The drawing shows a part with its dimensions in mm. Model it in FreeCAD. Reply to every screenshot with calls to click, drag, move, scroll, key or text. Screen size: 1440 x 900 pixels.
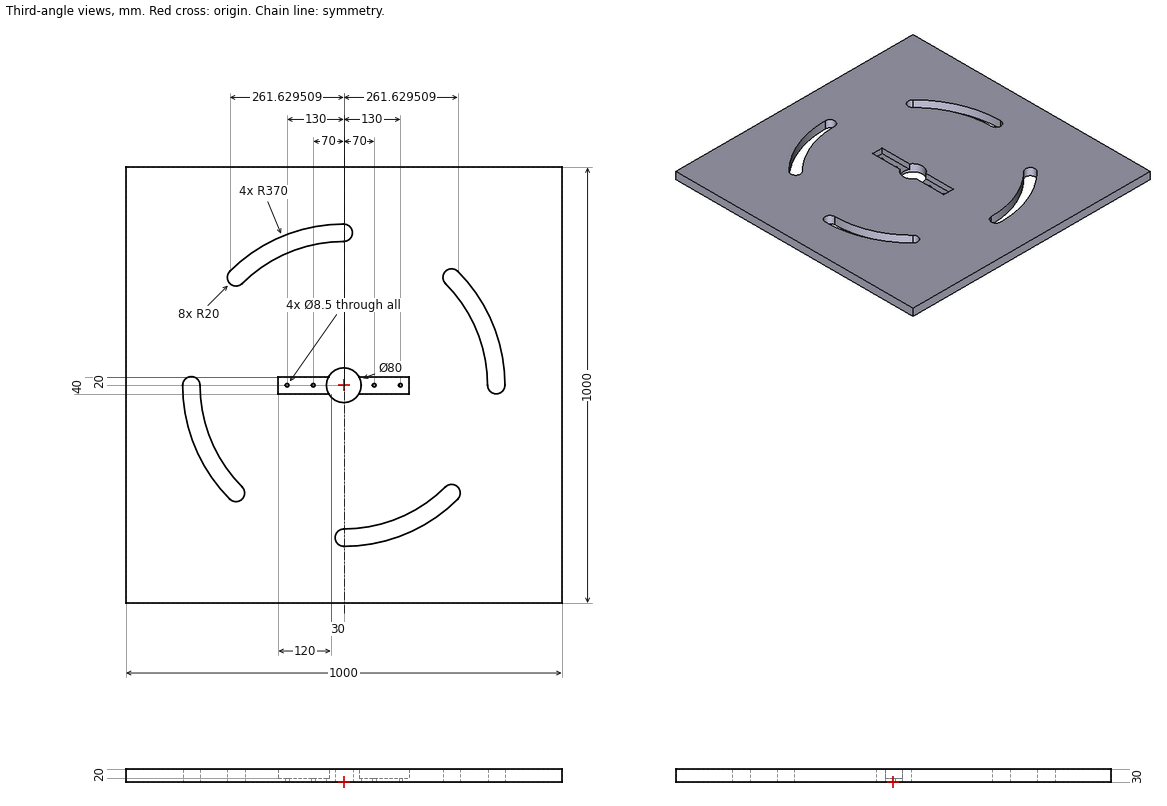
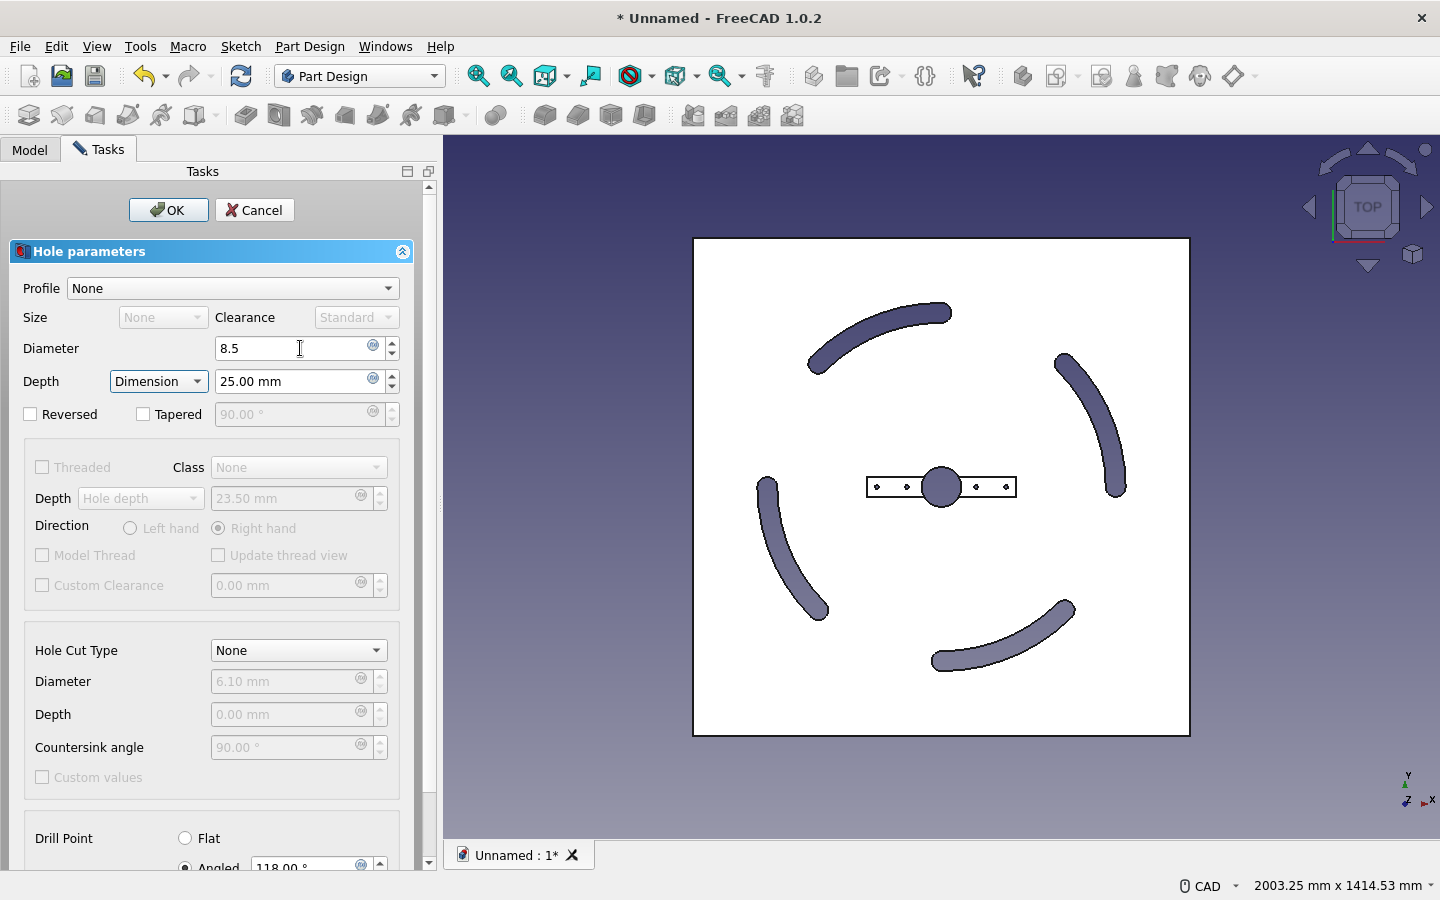
click(160, 382)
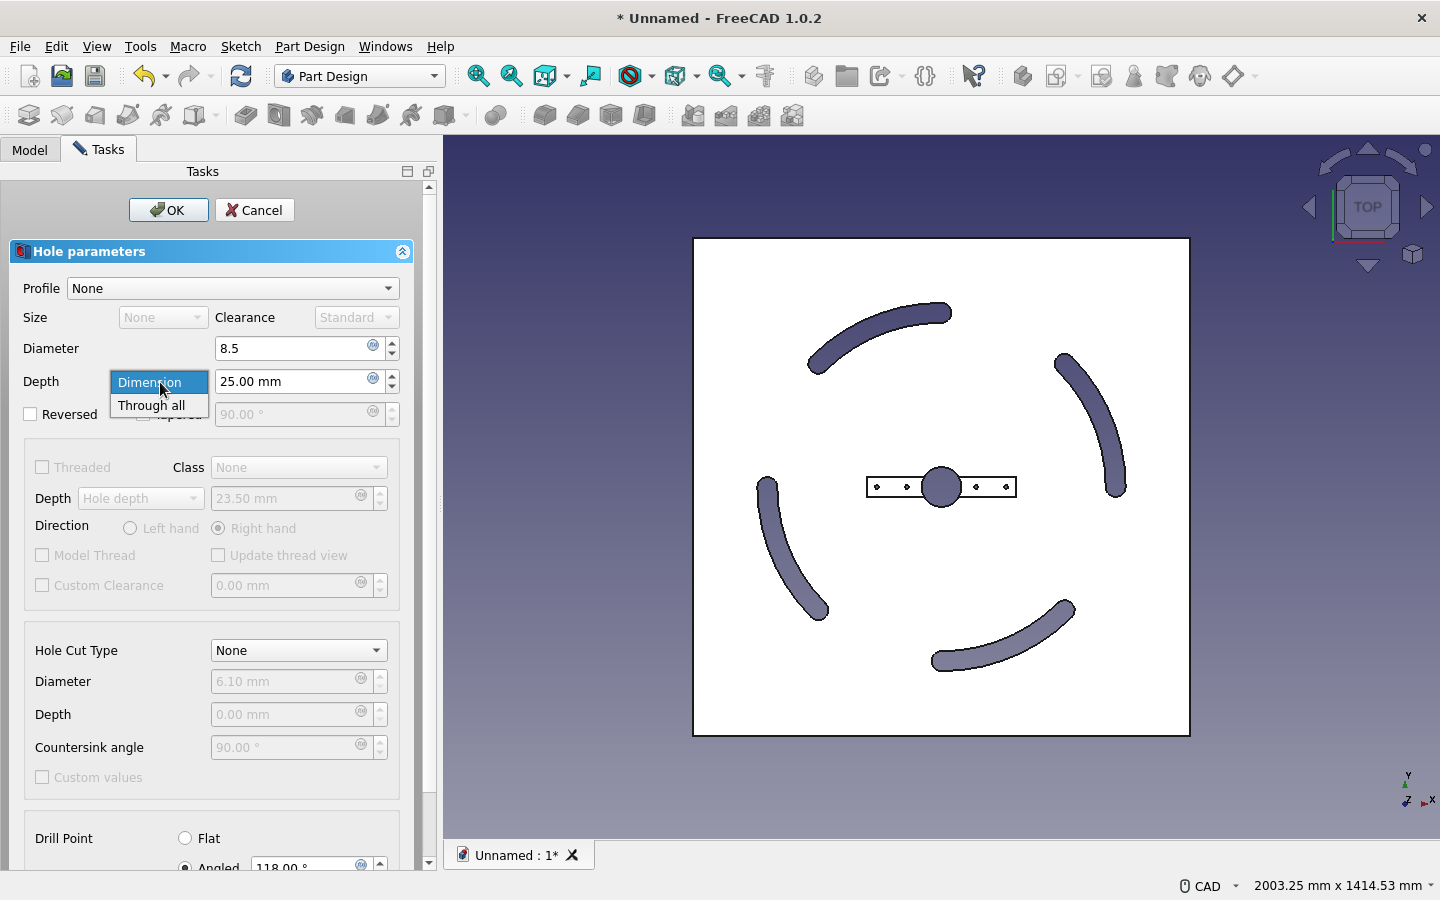
click(158, 406)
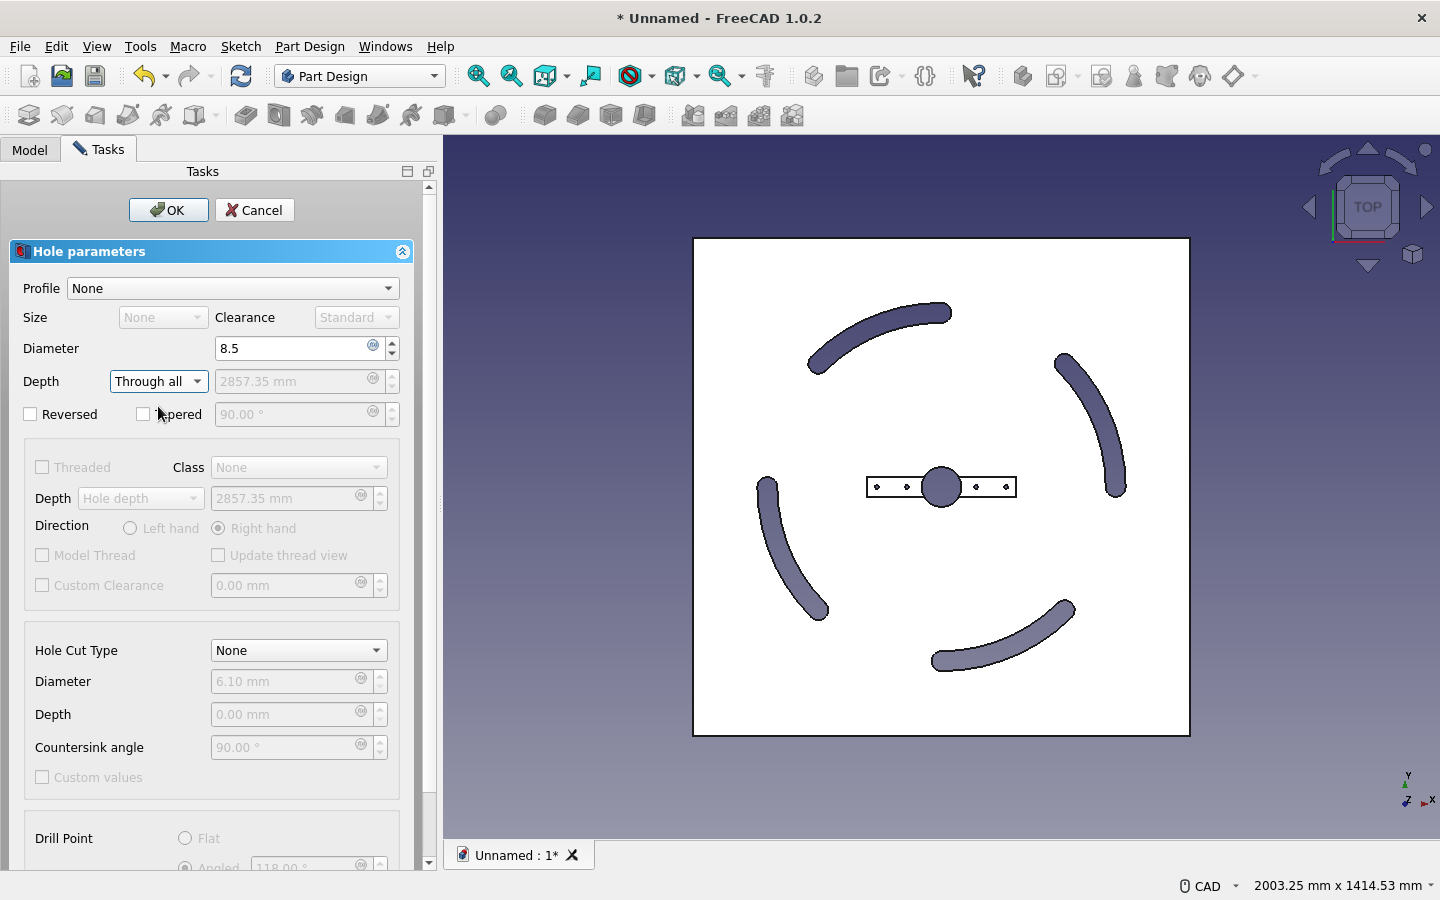
click(169, 210)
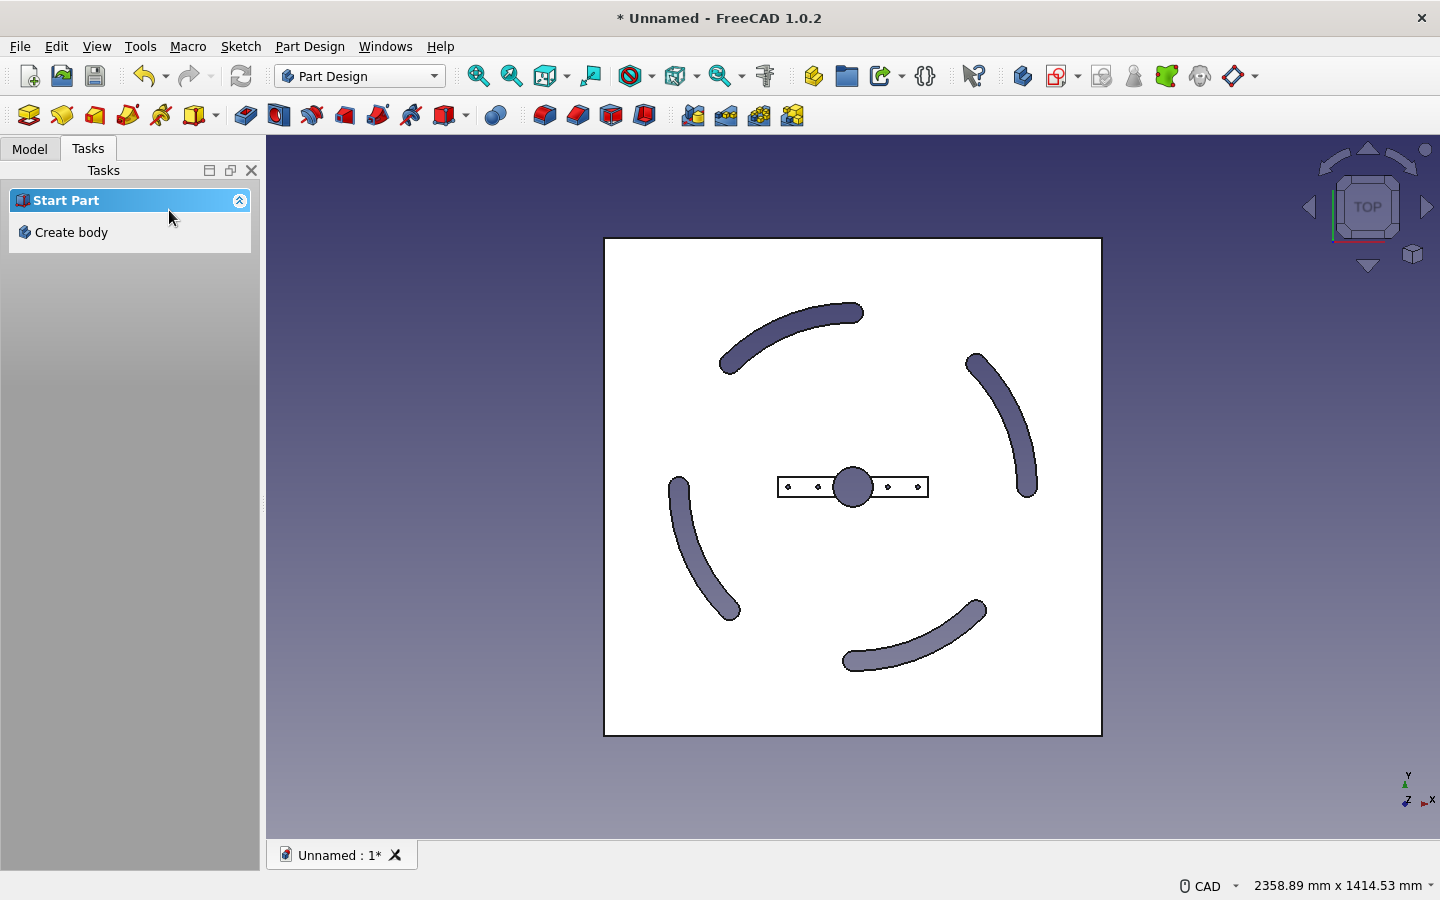
key(0)